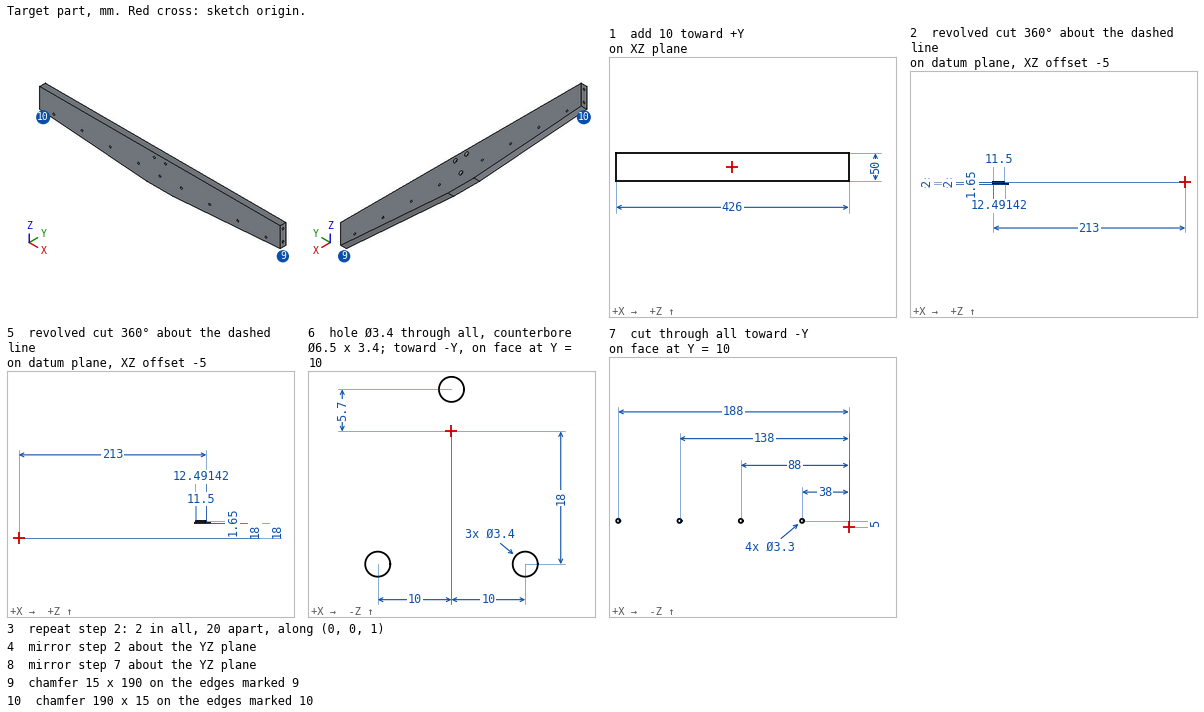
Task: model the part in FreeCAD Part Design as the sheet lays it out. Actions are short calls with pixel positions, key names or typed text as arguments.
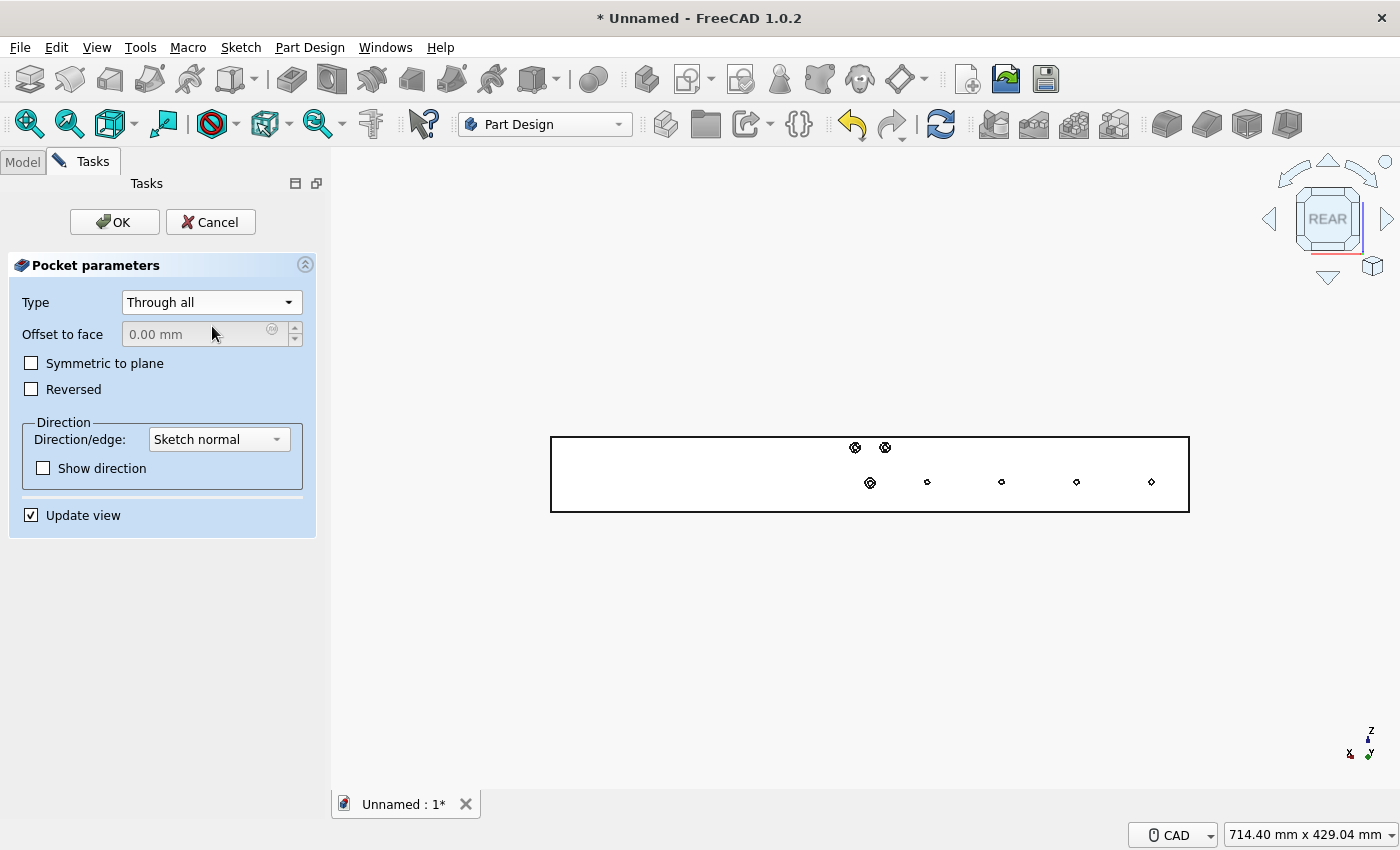
click(115, 222)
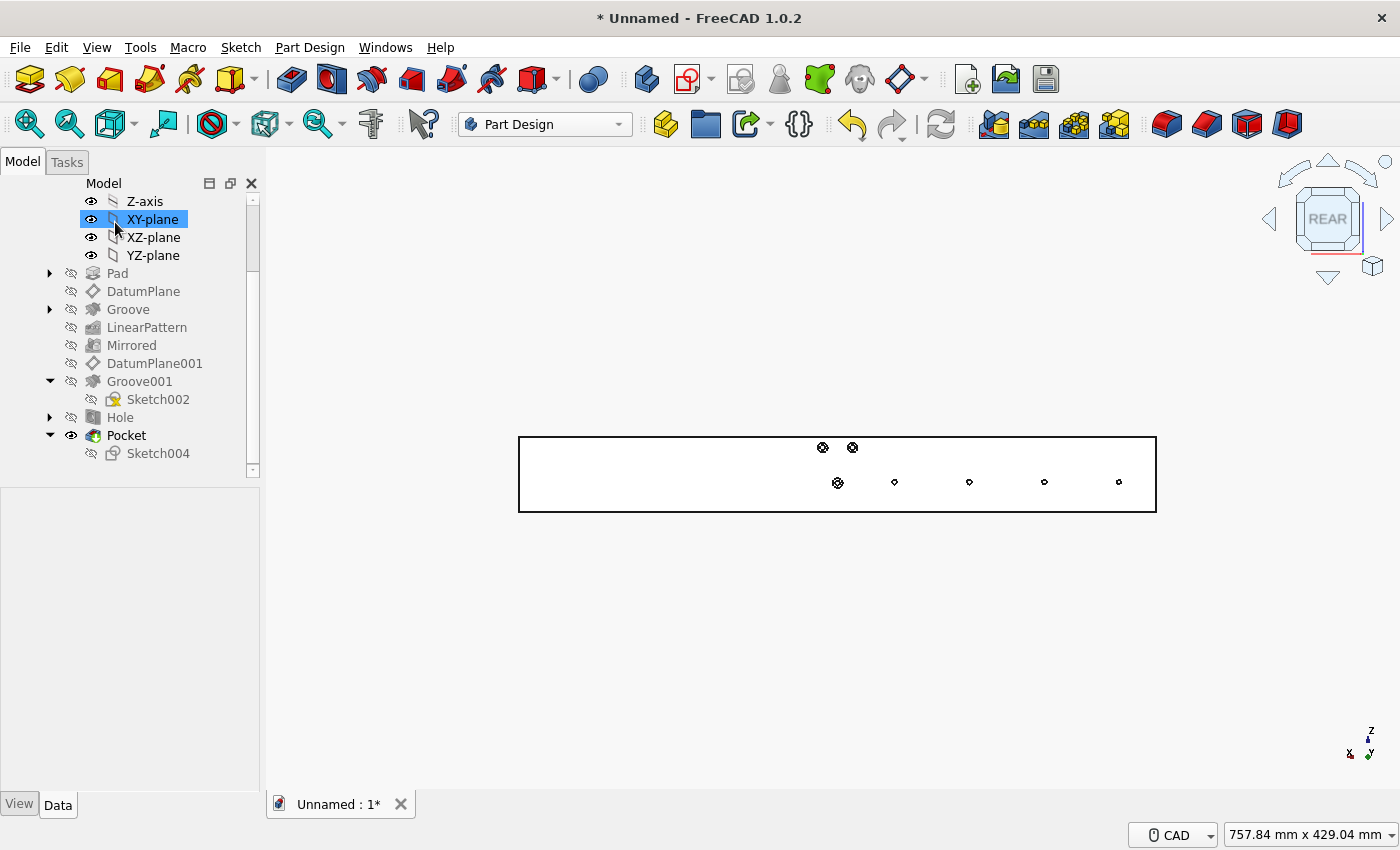
click(116, 435)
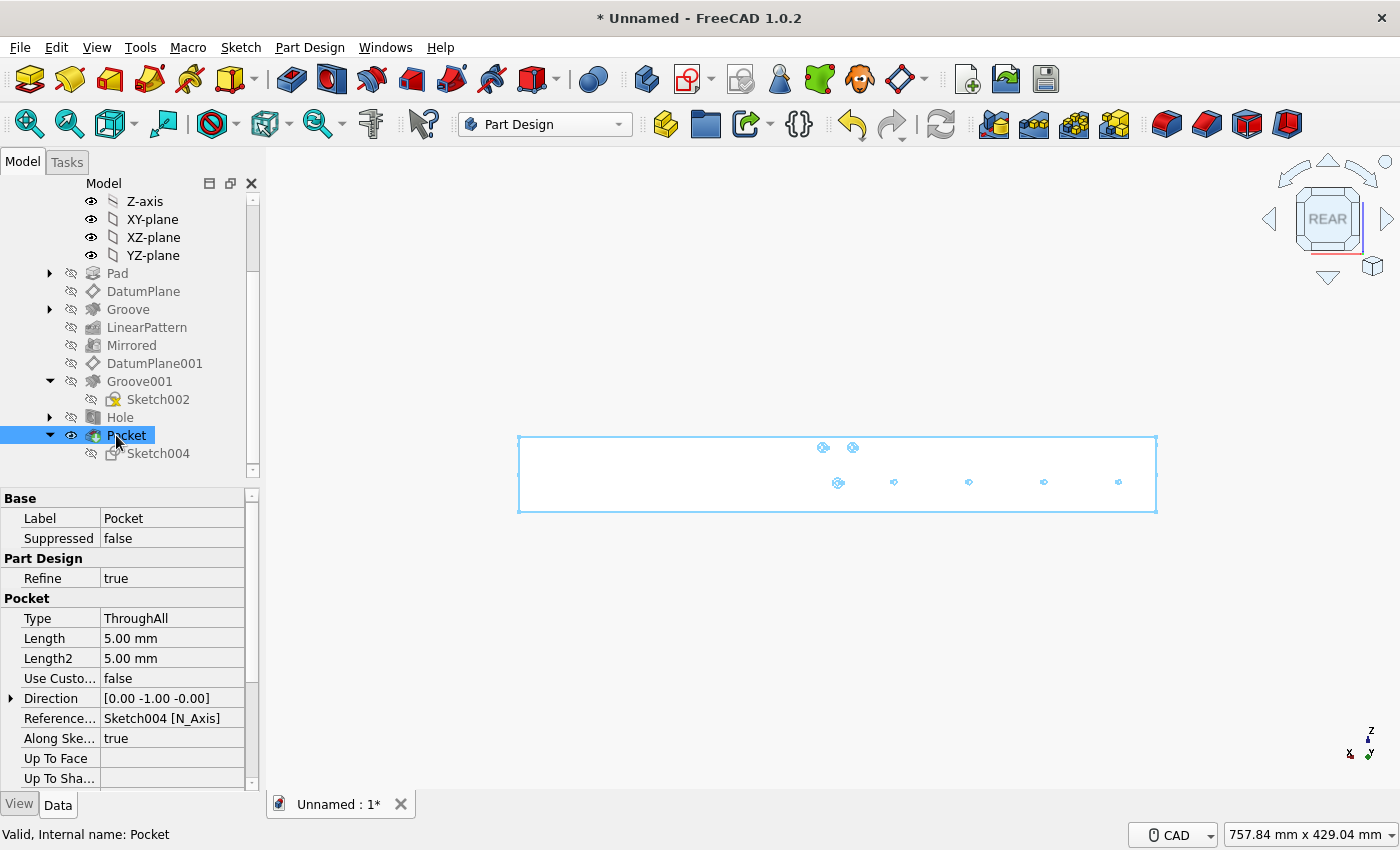
click(994, 124)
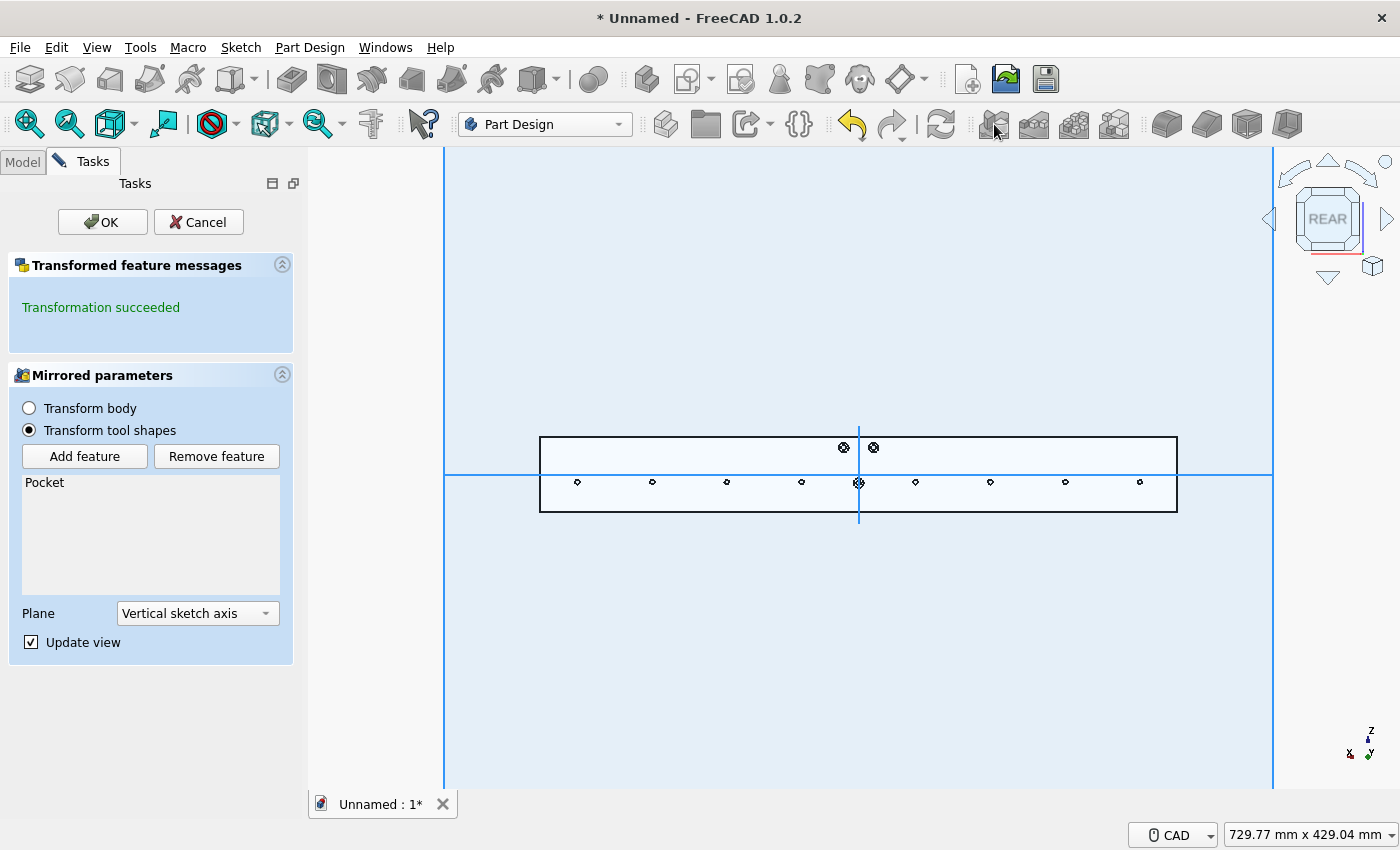
click(198, 614)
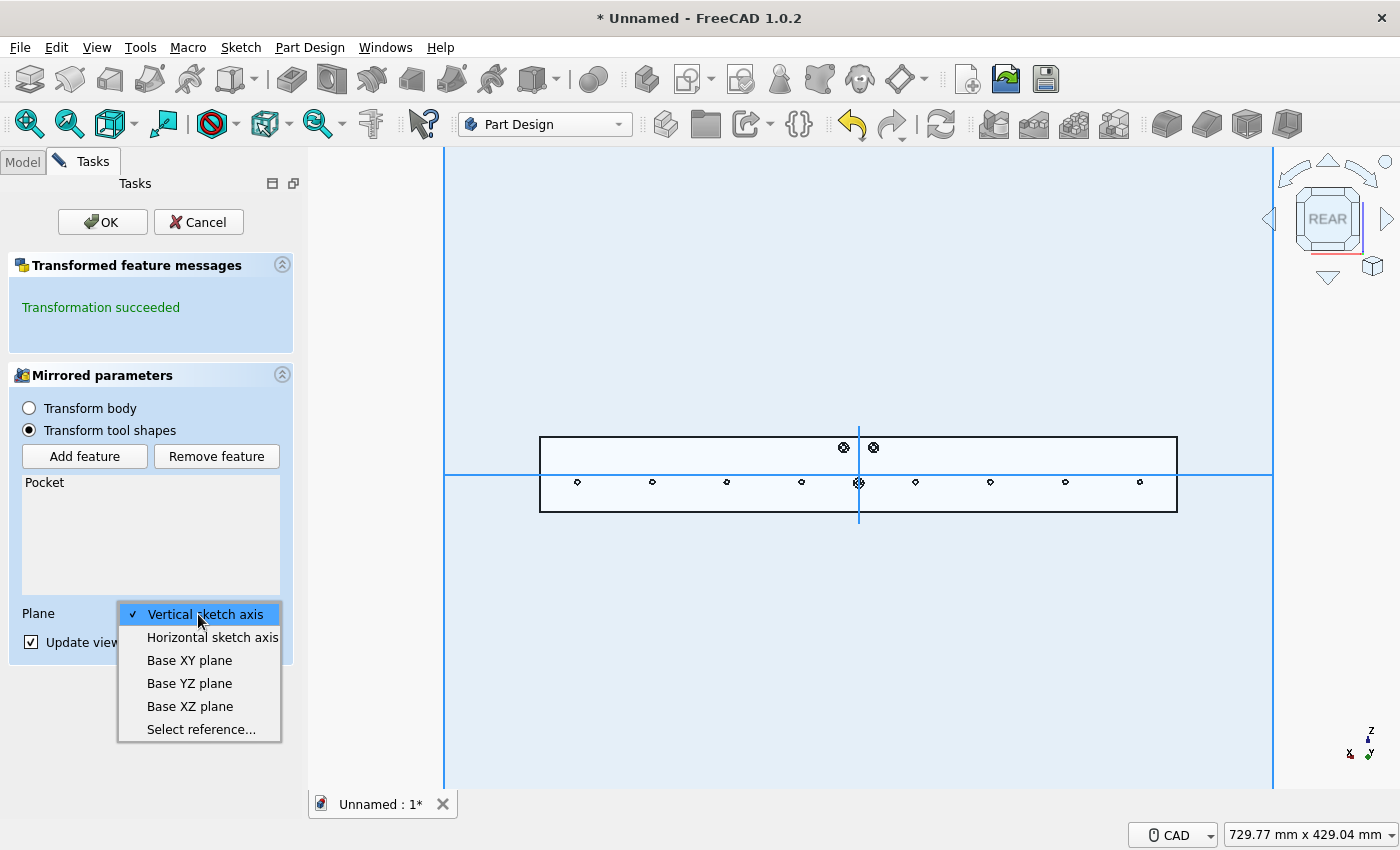
click(198, 684)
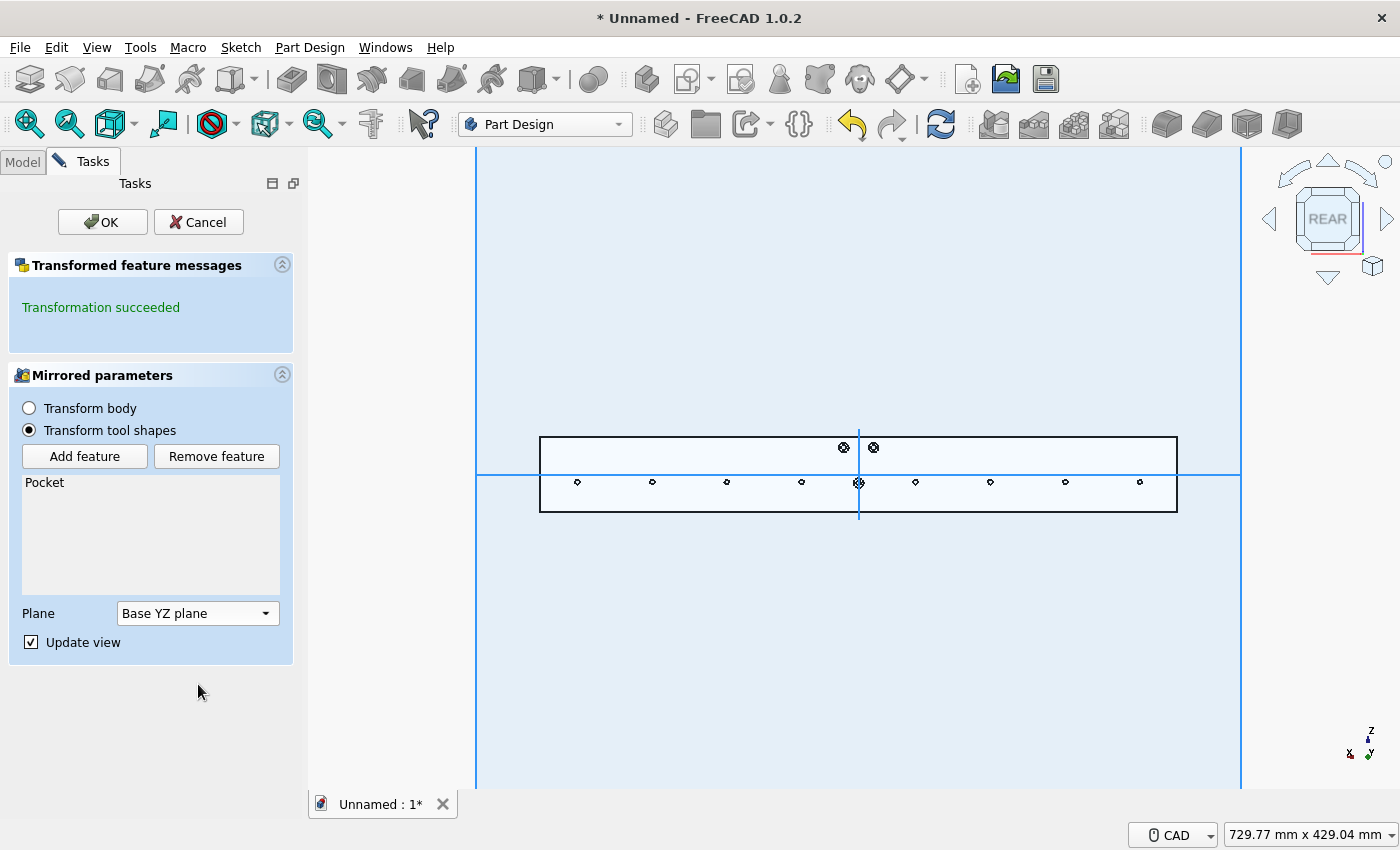
click(103, 222)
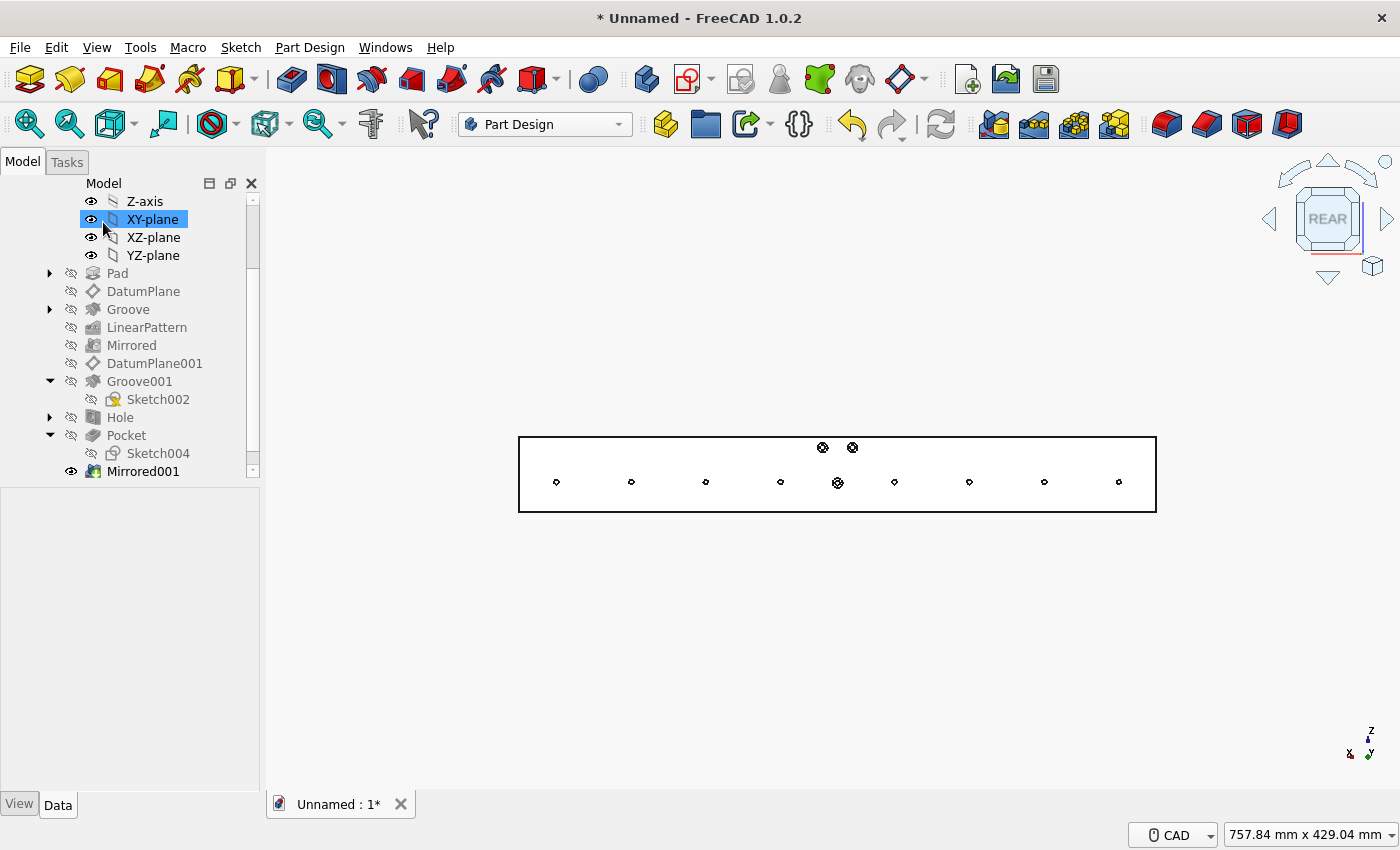
scroll(519, 511, up, 5)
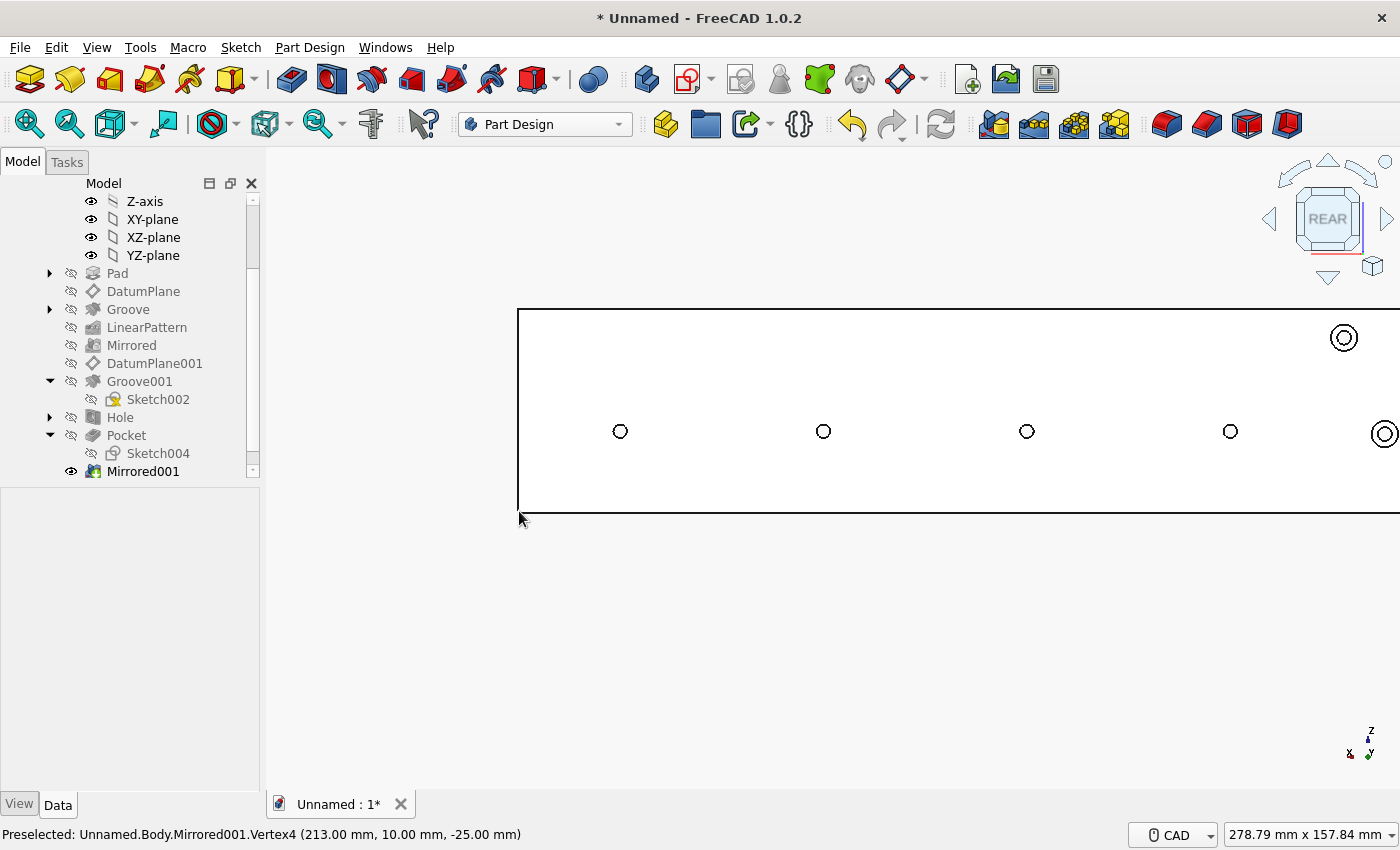
click(30, 124)